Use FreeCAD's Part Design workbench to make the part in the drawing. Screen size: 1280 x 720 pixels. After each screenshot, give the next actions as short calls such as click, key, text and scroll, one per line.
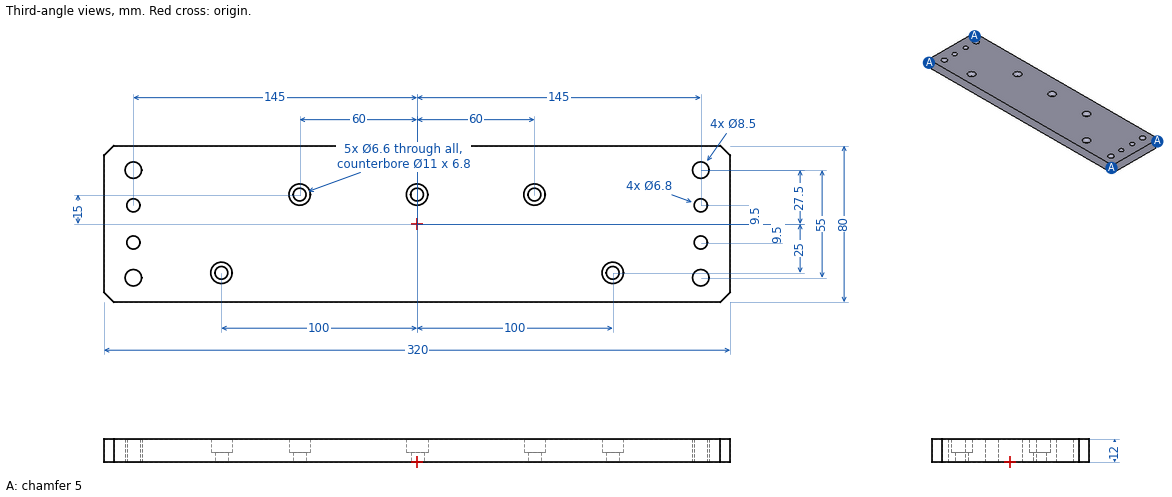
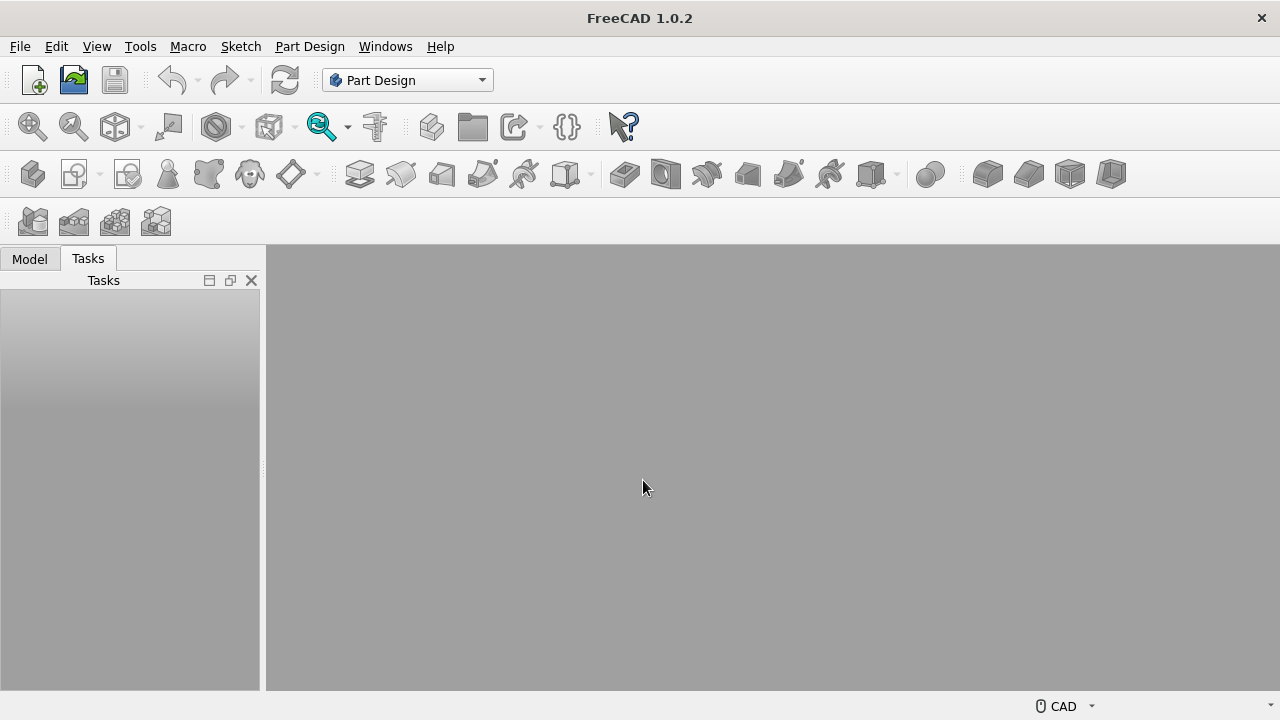
click(33, 80)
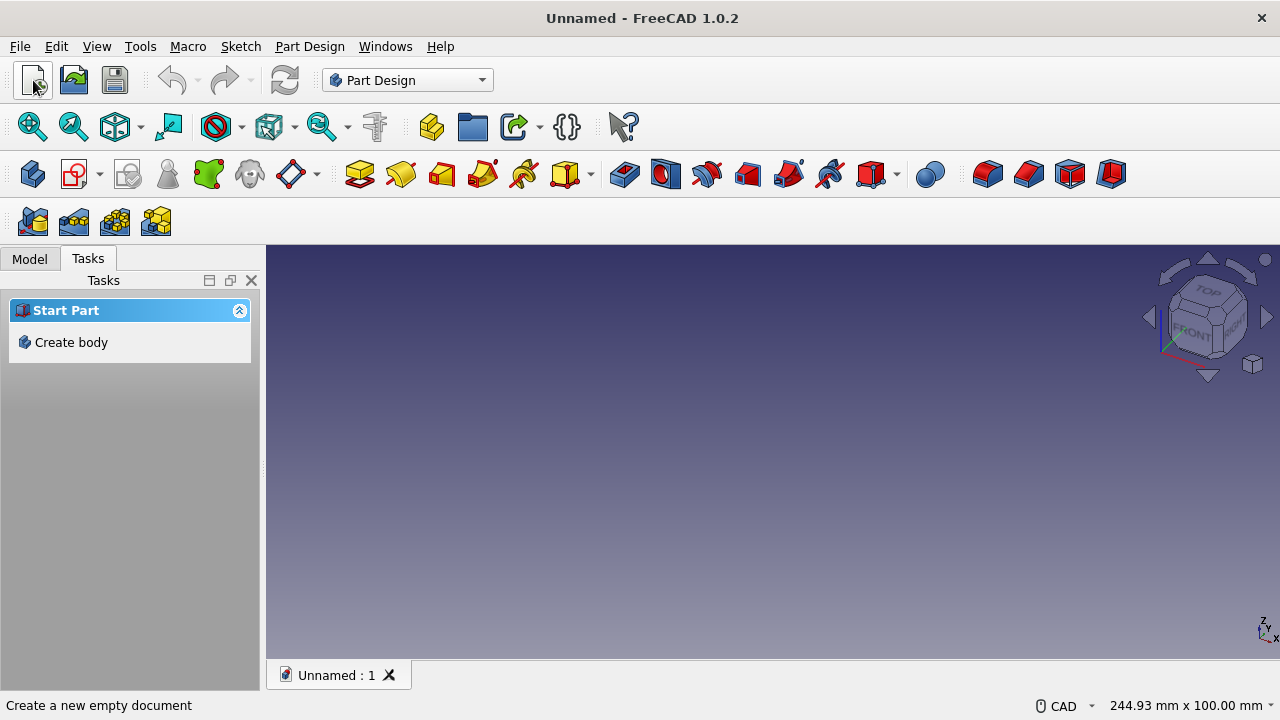
click(74, 174)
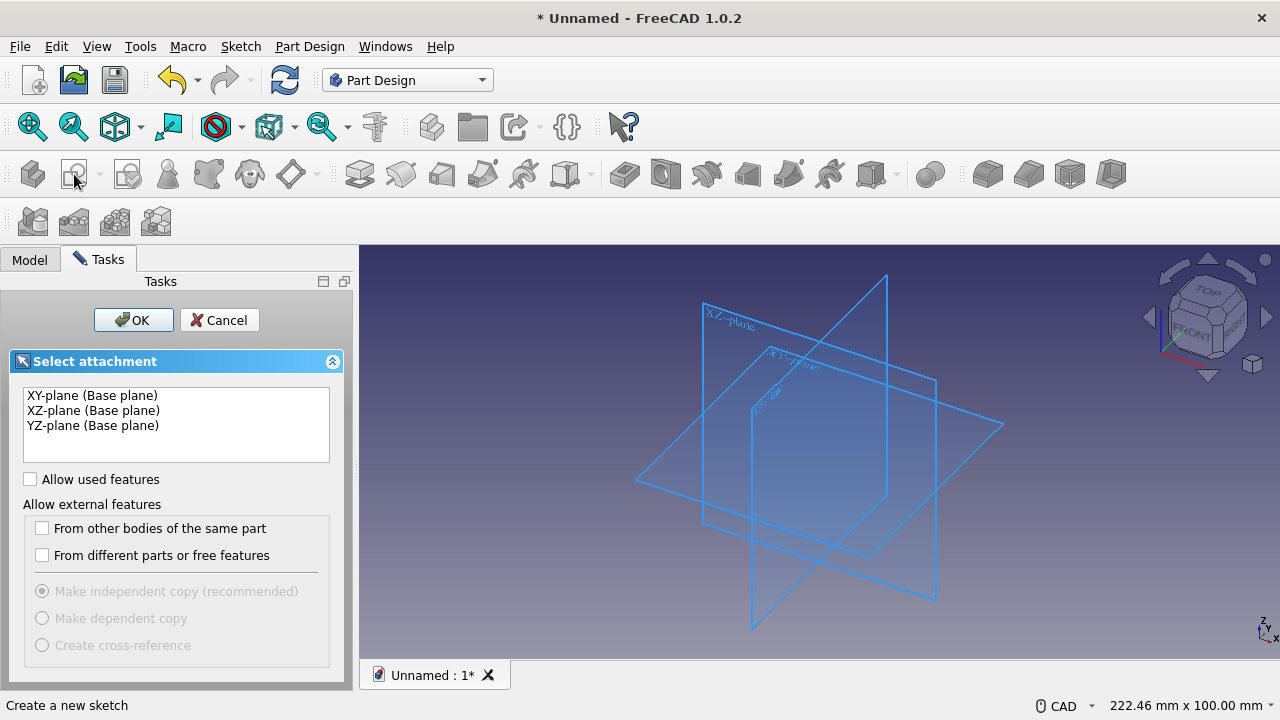
click(84, 396)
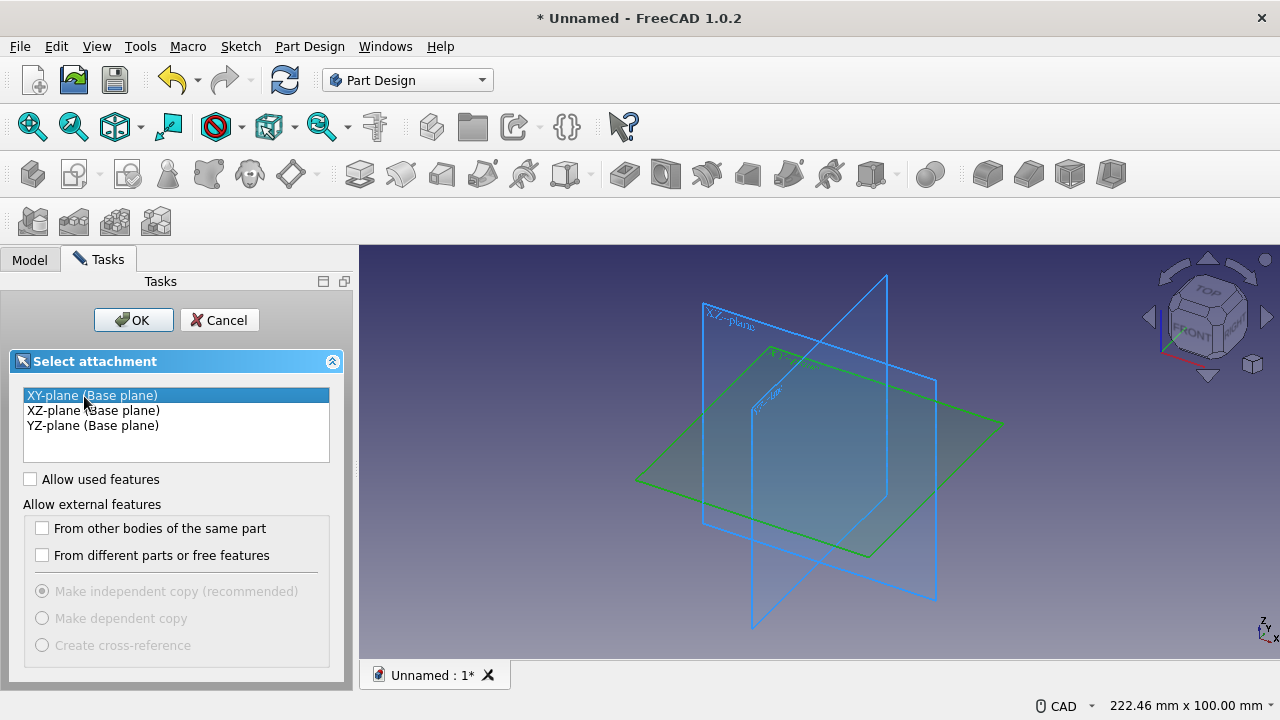
click(134, 320)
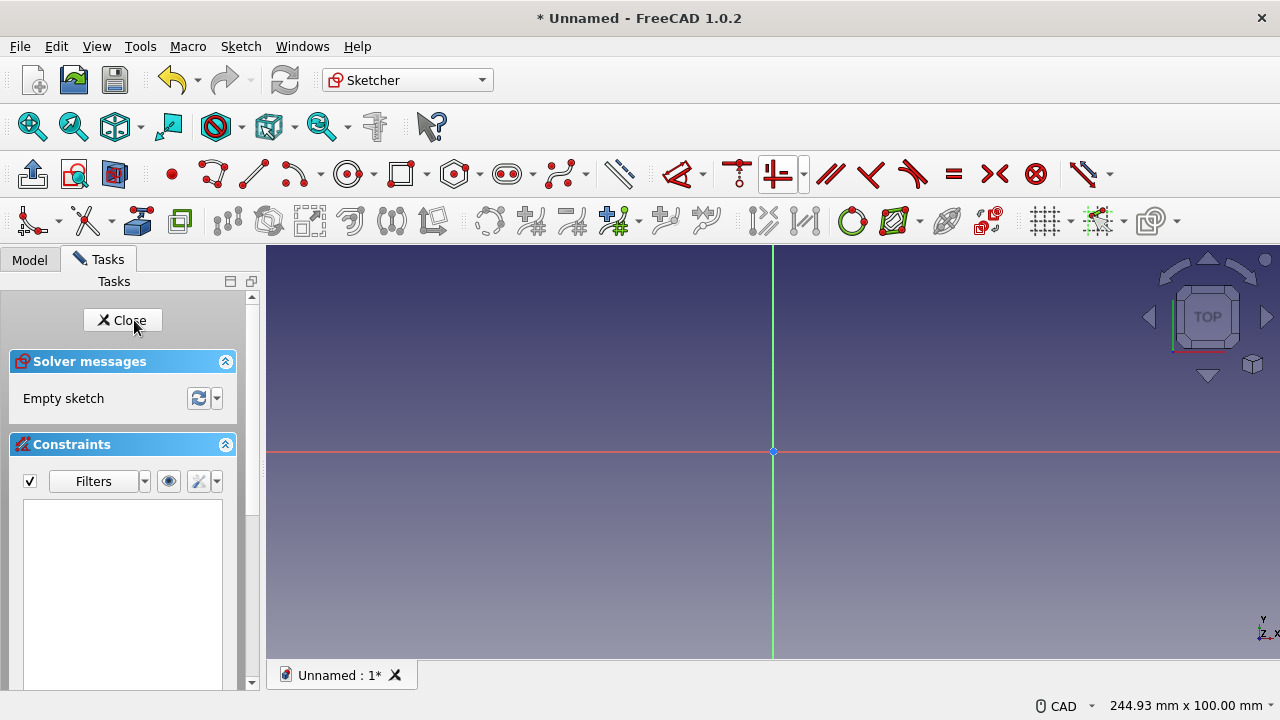
scroll(649, 452, down, 4)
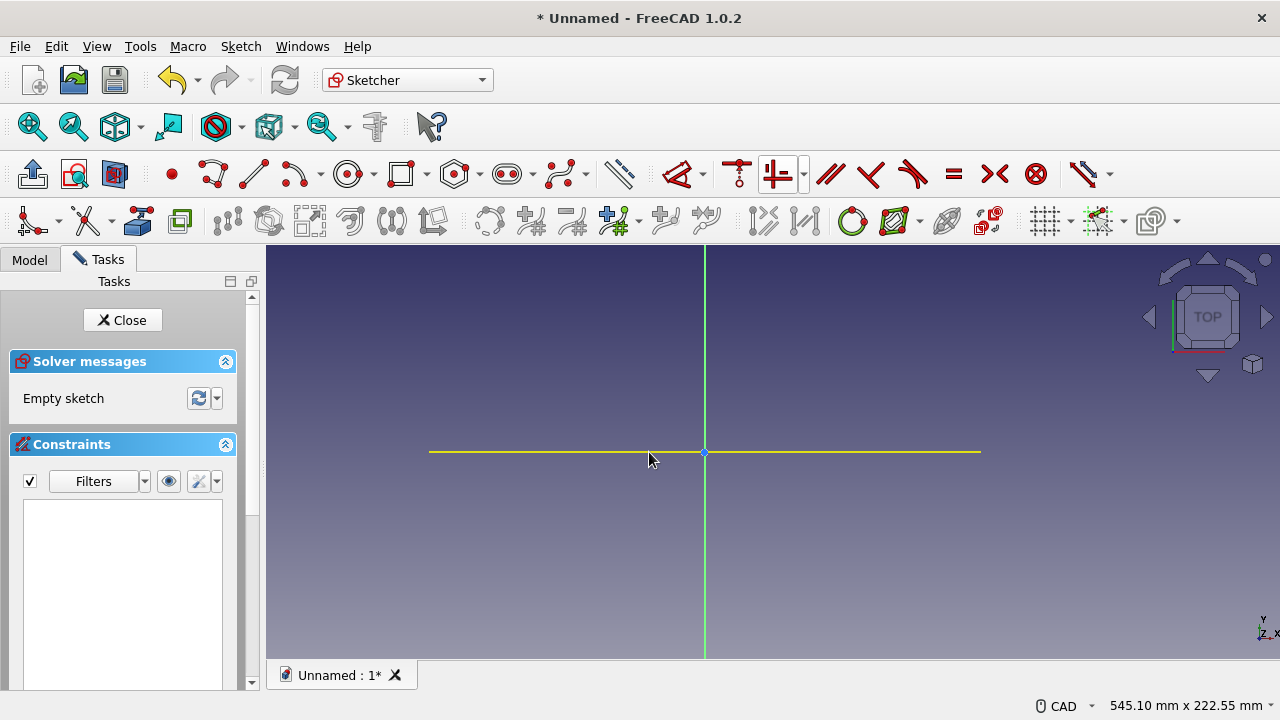
key(g)
key(v)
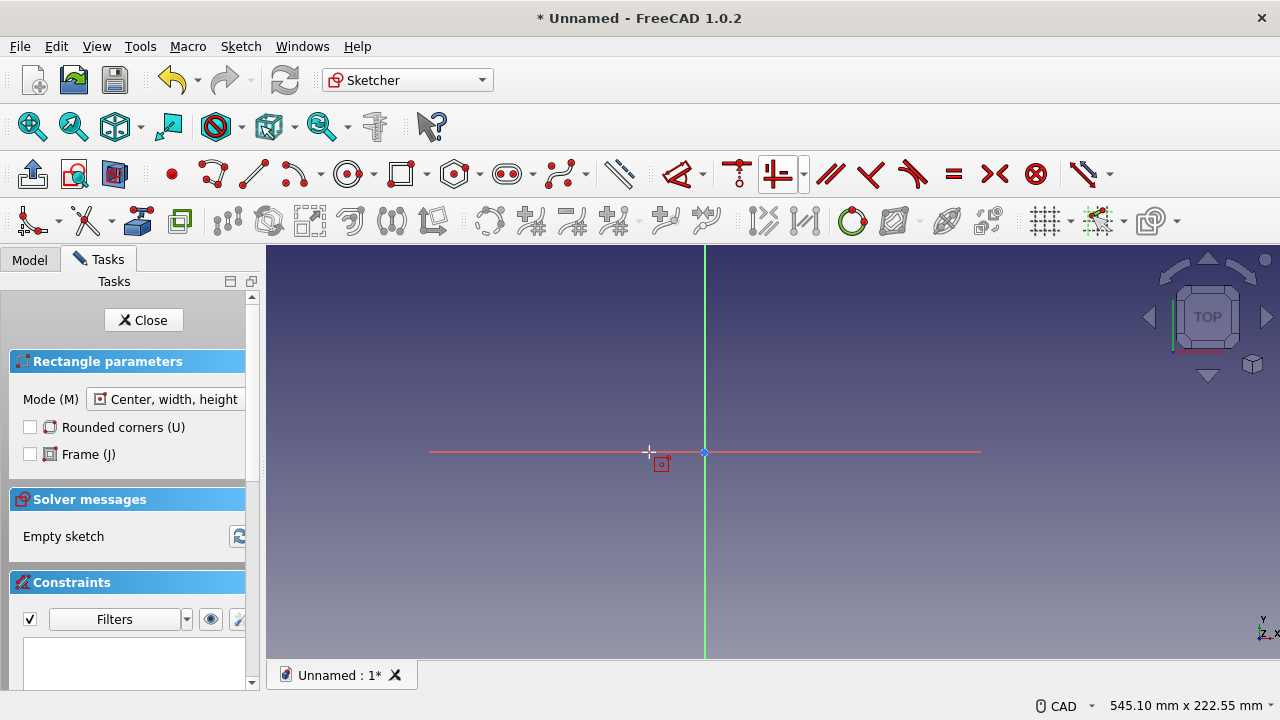
click(705, 452)
click(1003, 378)
key(Escape)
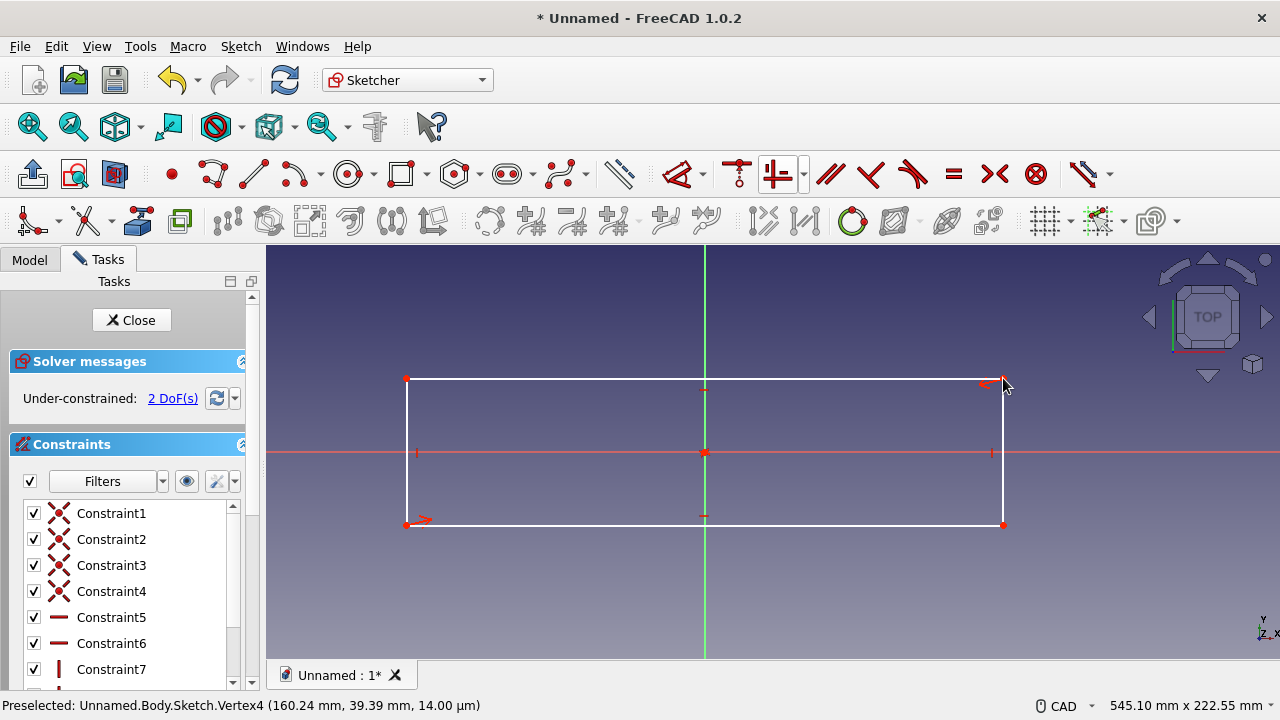
click(676, 174)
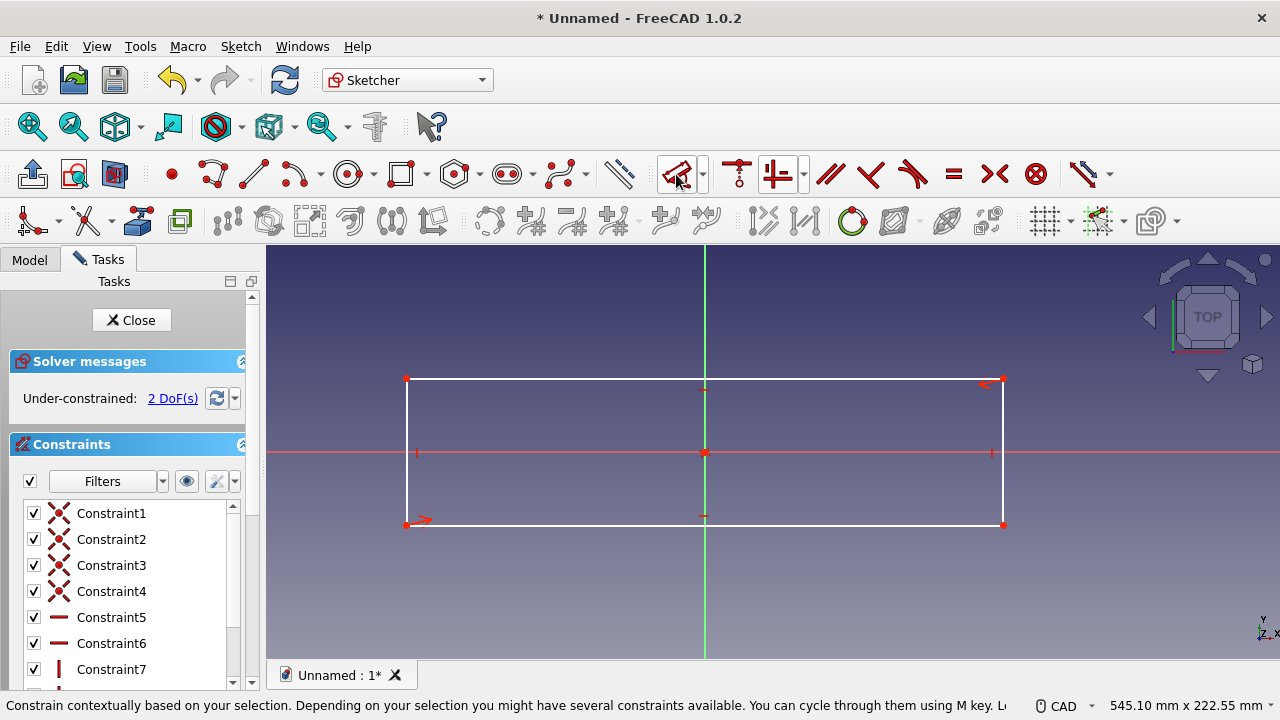
click(1003, 482)
click(1037, 419)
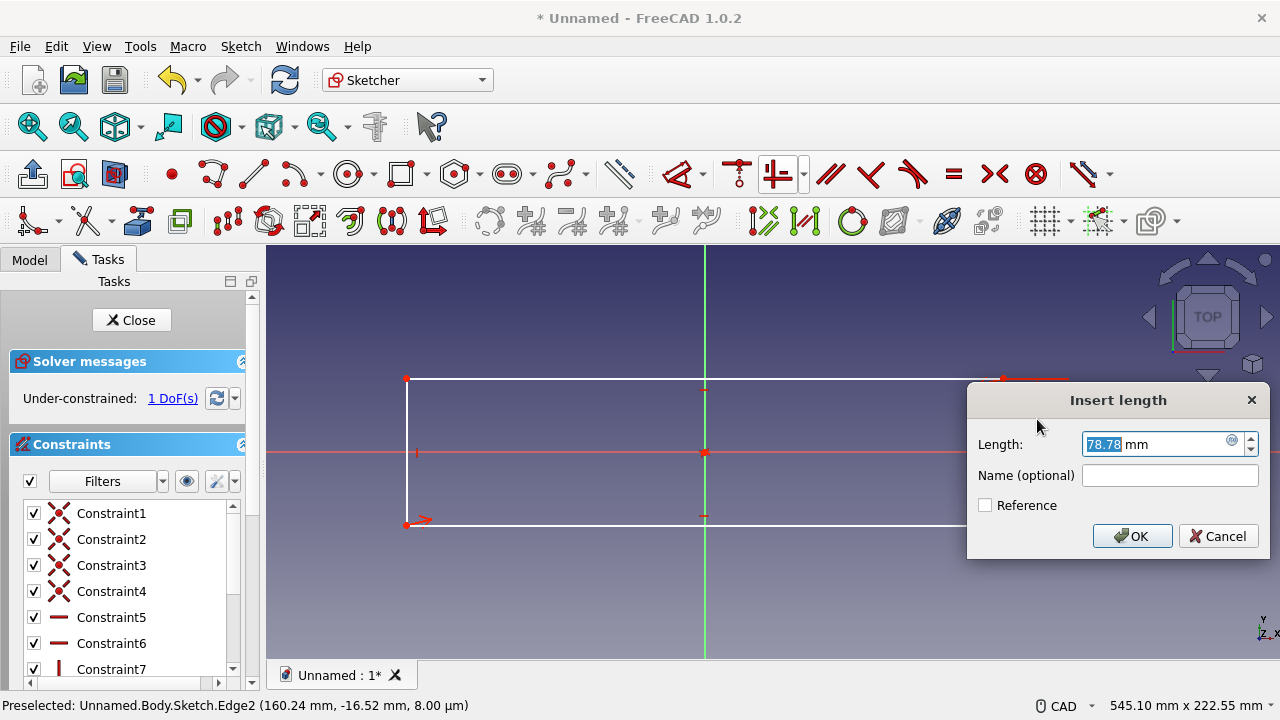
text(80)
key(Return)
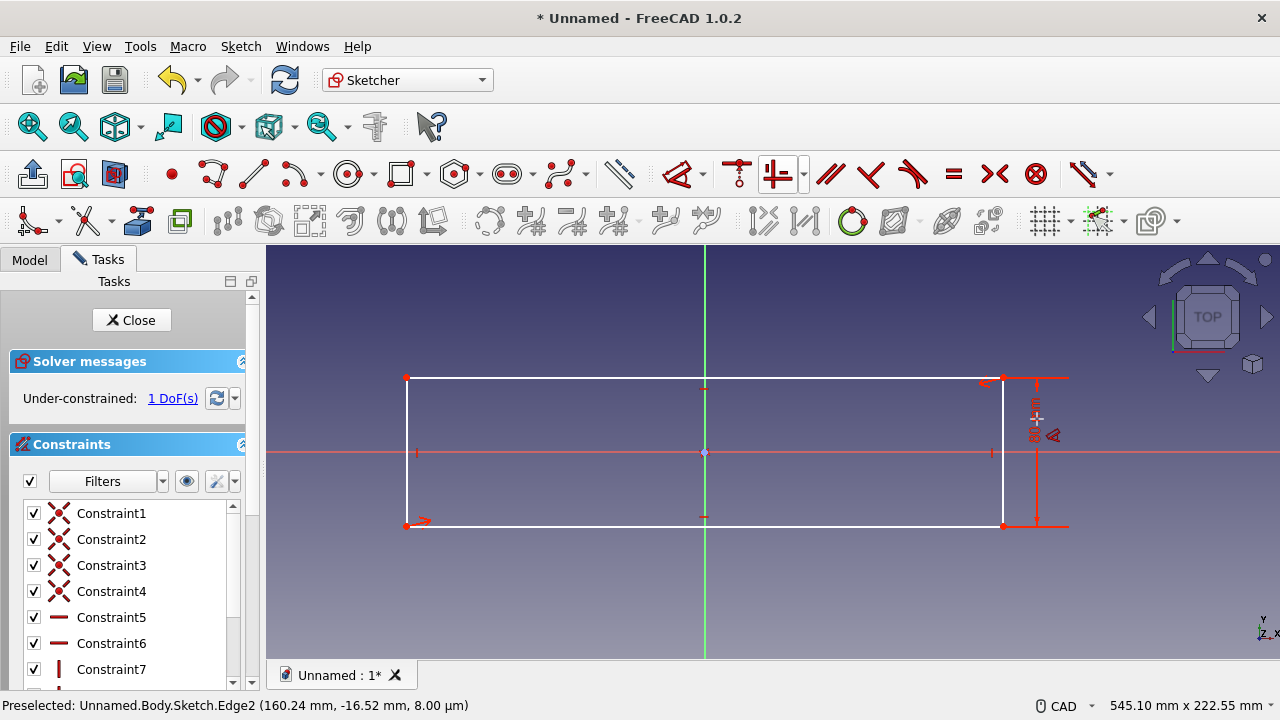
click(586, 527)
click(568, 561)